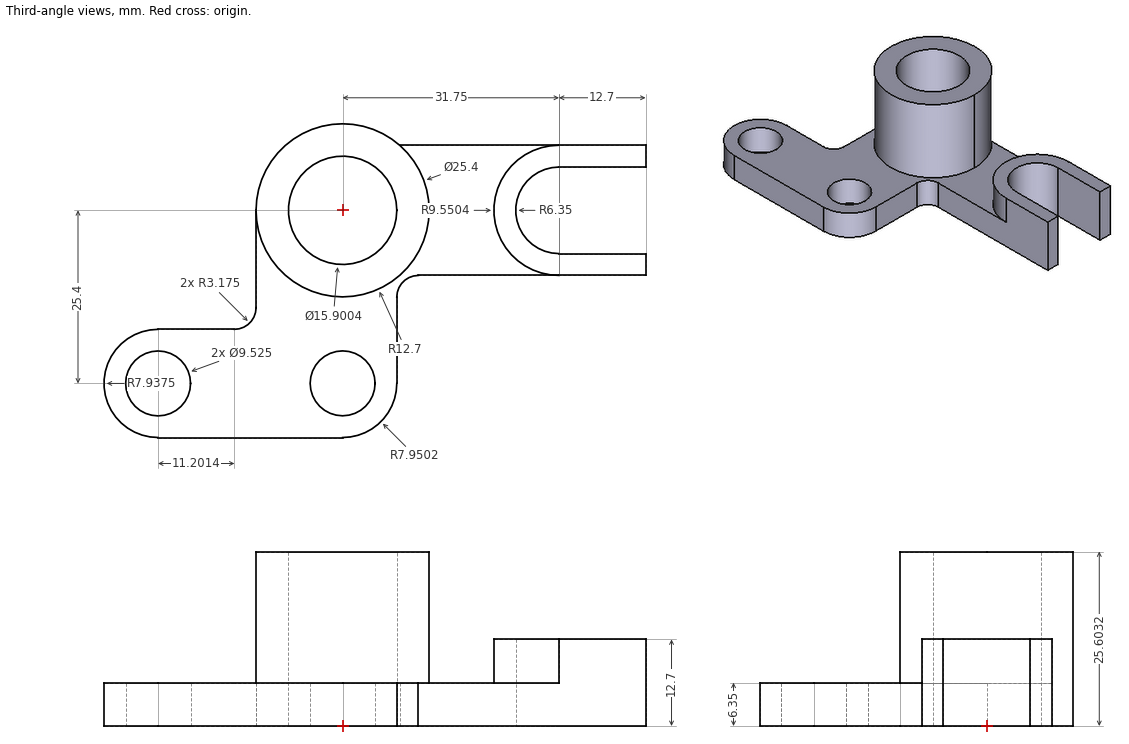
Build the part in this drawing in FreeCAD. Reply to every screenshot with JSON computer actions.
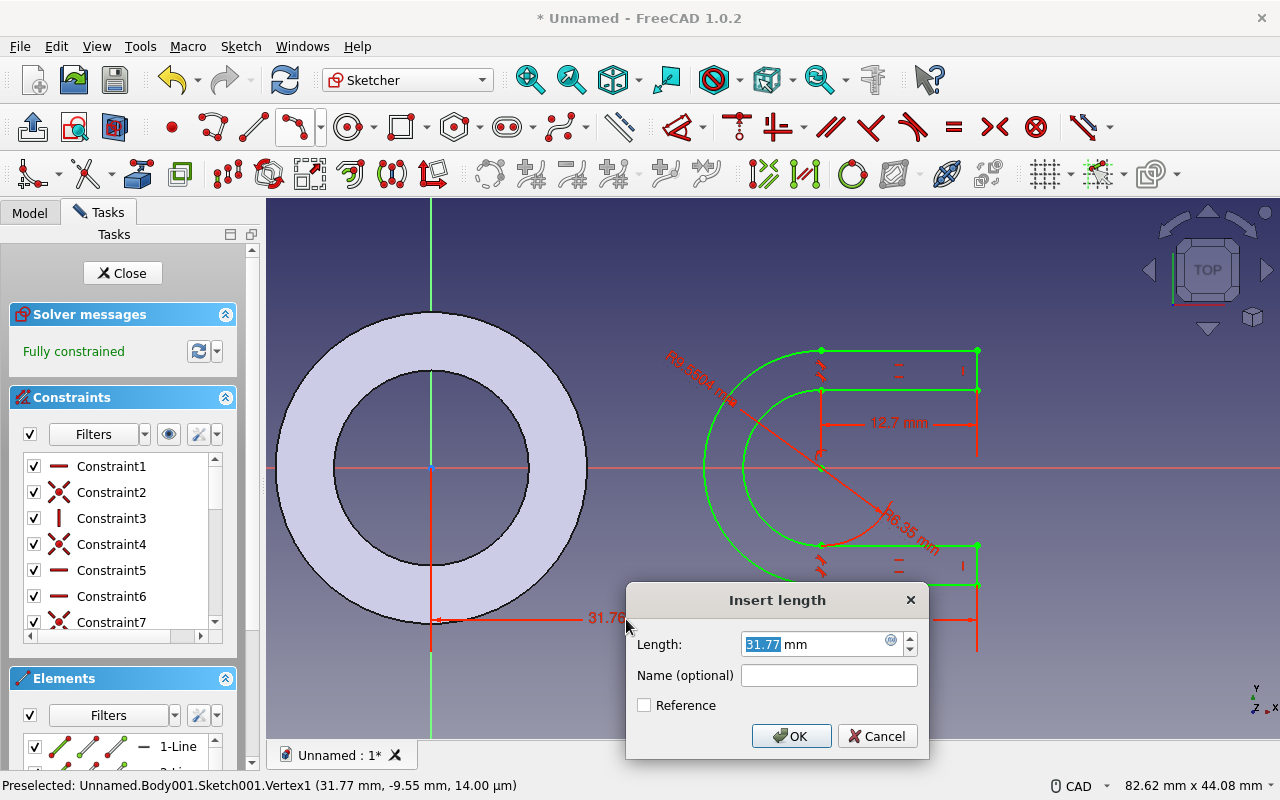
{"action": "type", "text": "31.75"}
{"action": "key", "text": "Return"}
{"action": "key", "text": "Escape"}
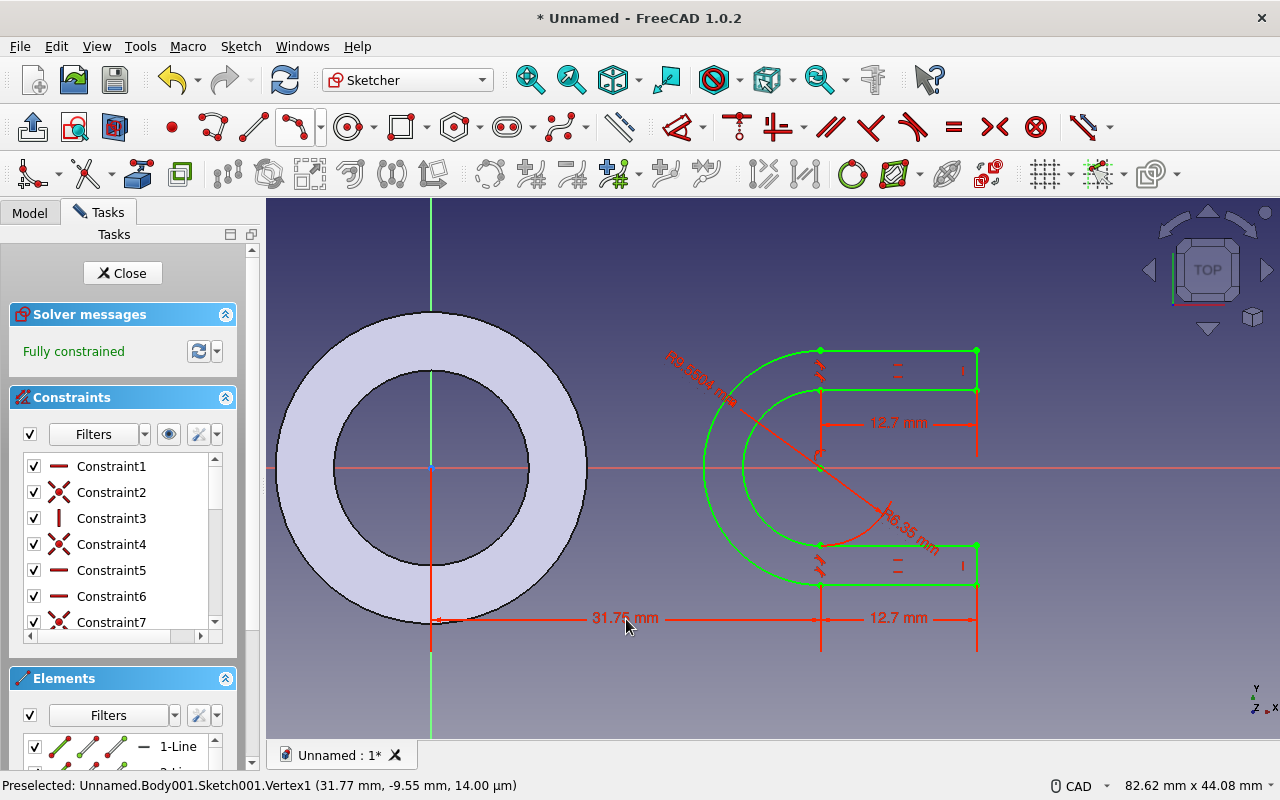
{"action": "left_click", "coordinate": [123, 273]}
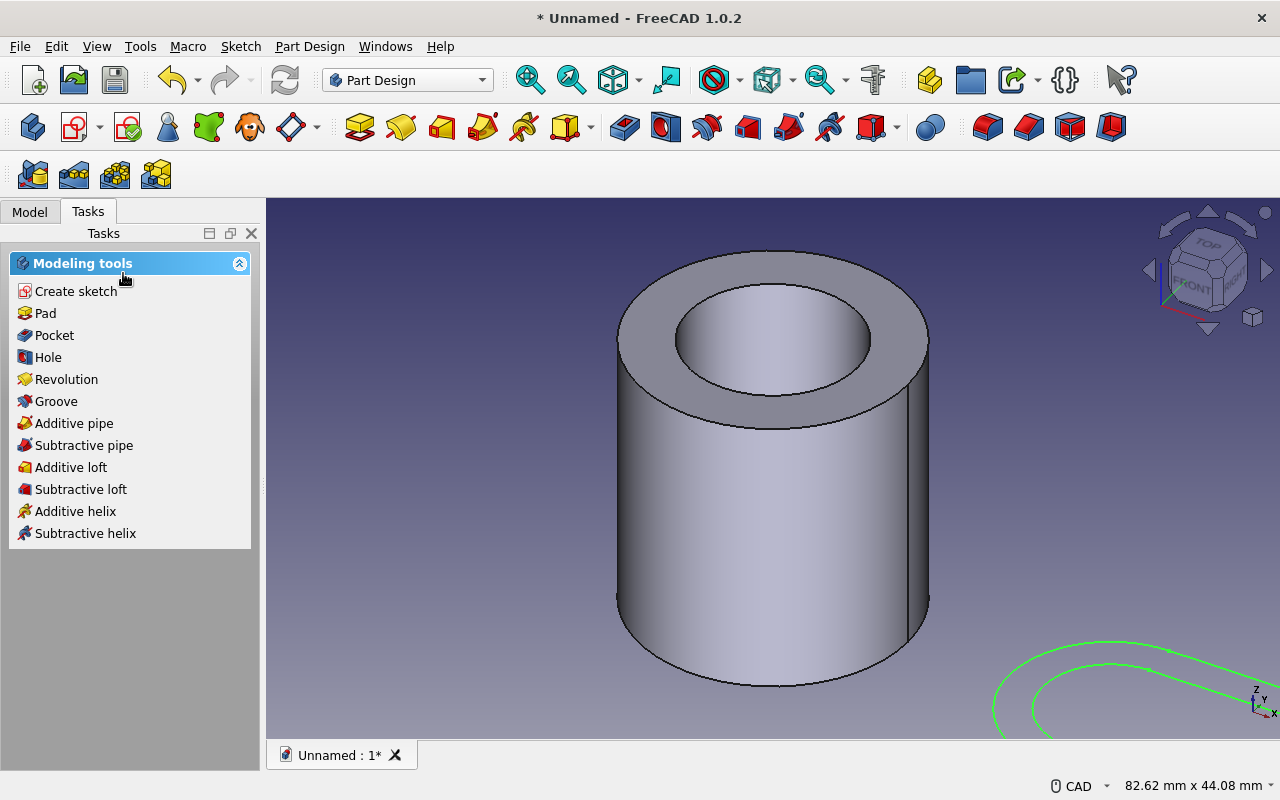
{"action": "left_click", "coordinate": [360, 128]}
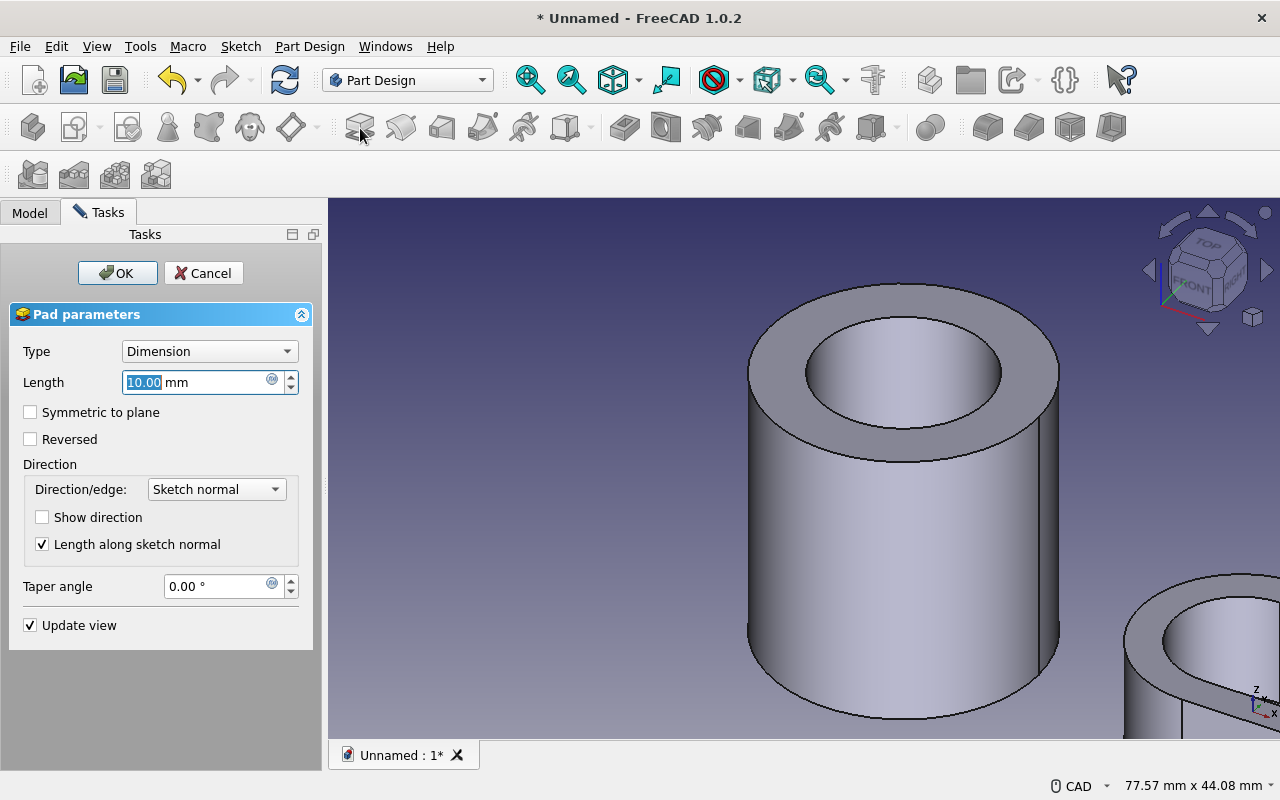
{"action": "type", "text": "12.7"}
{"action": "key", "text": "Tab"}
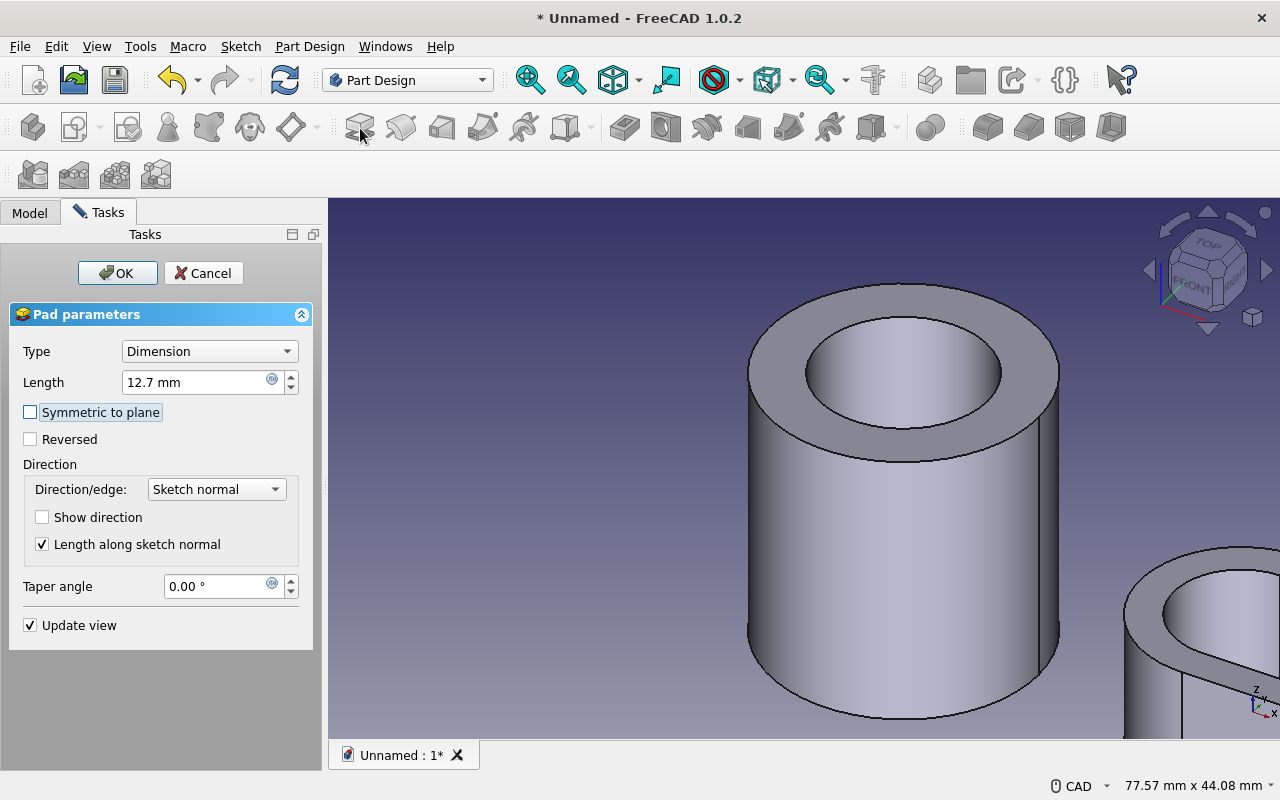
{"action": "left_click", "coordinate": [118, 273]}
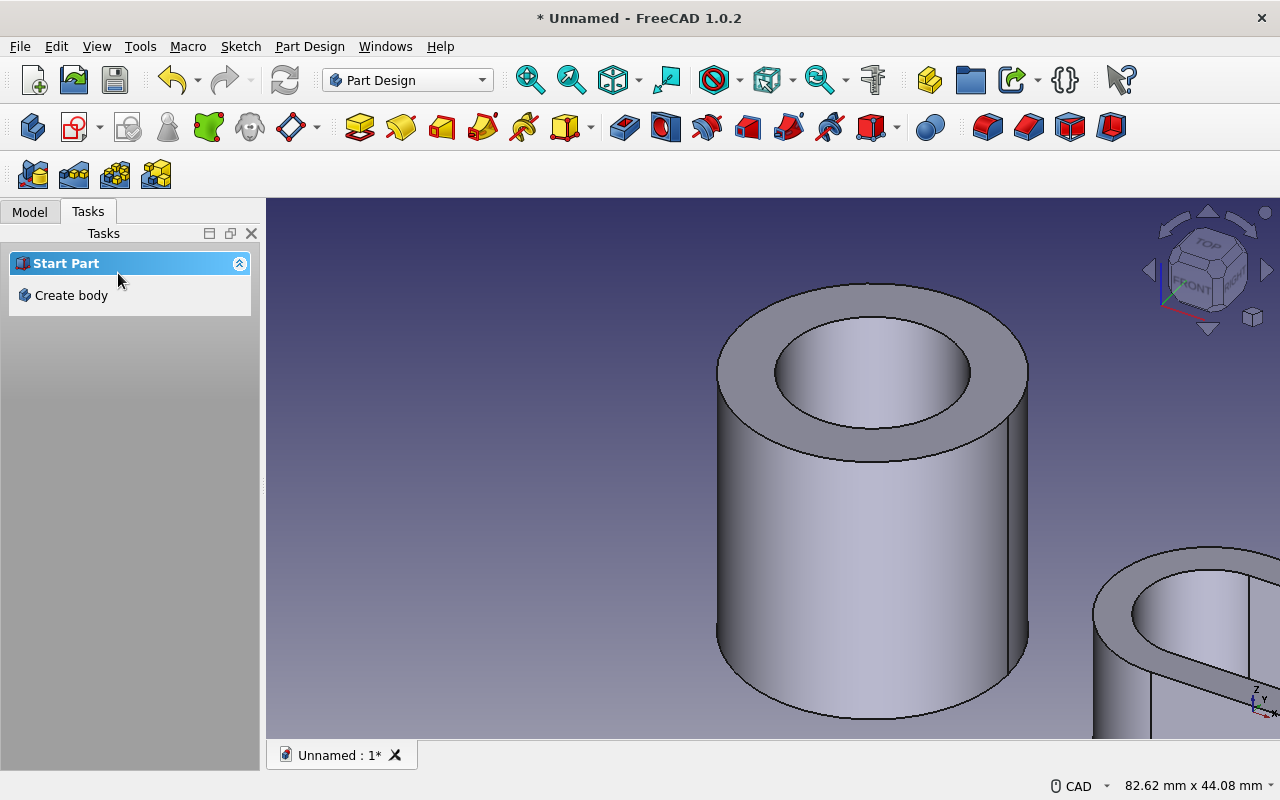
{"action": "left_click", "coordinate": [531, 80]}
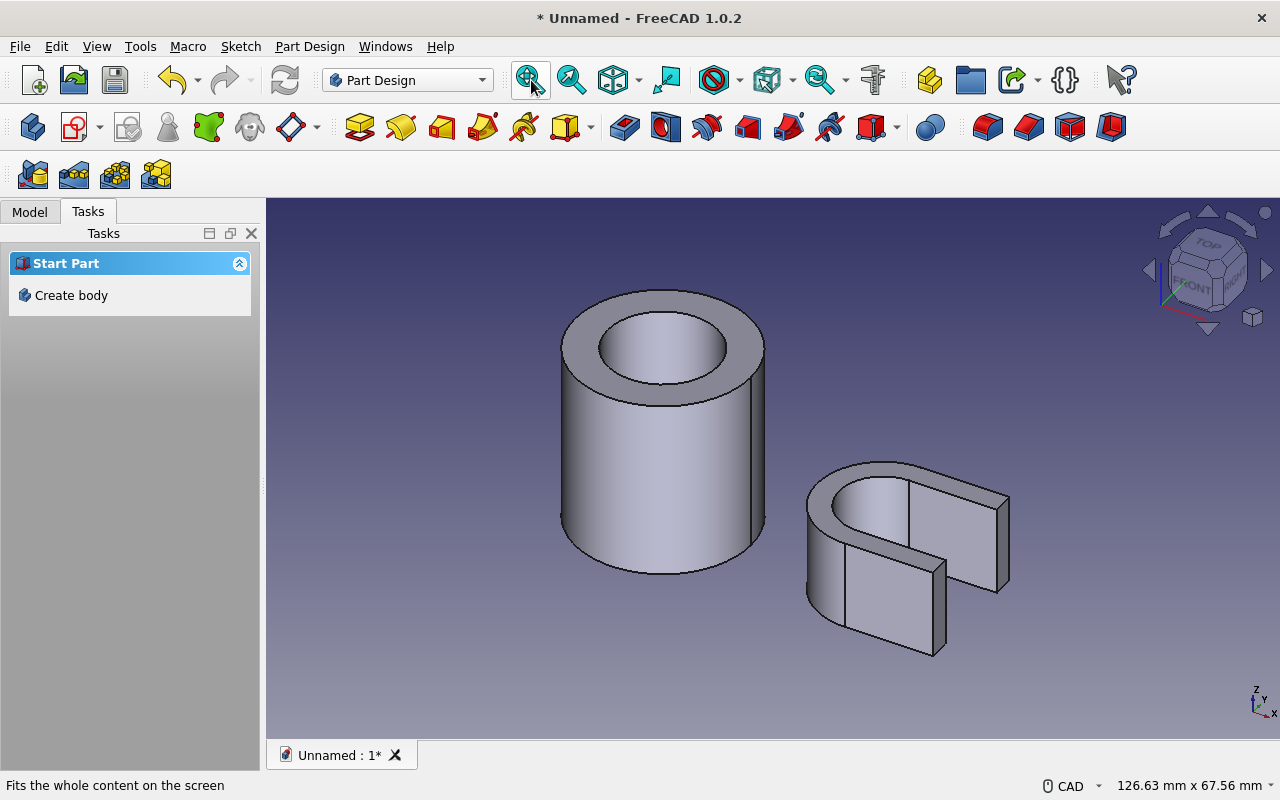
{"action": "left_click", "coordinate": [30, 212]}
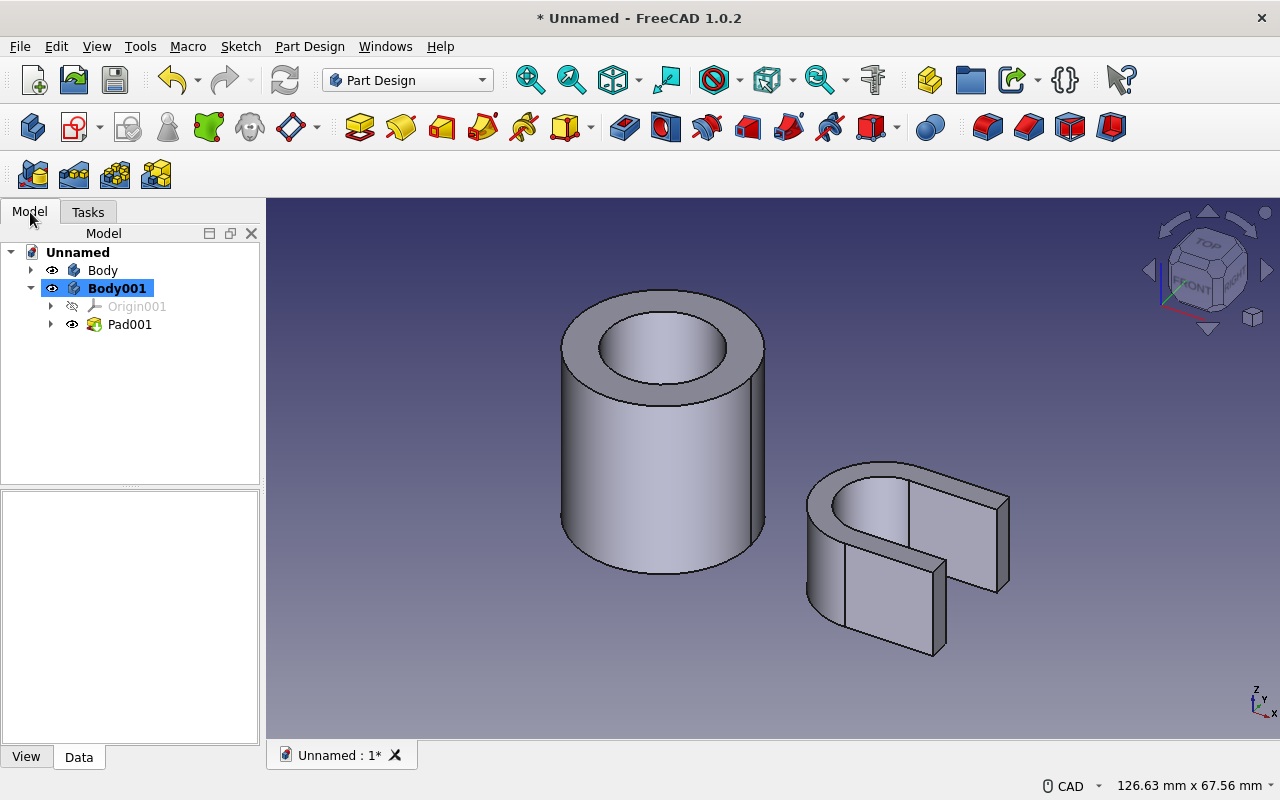
{"action": "double_click", "coordinate": [97, 270]}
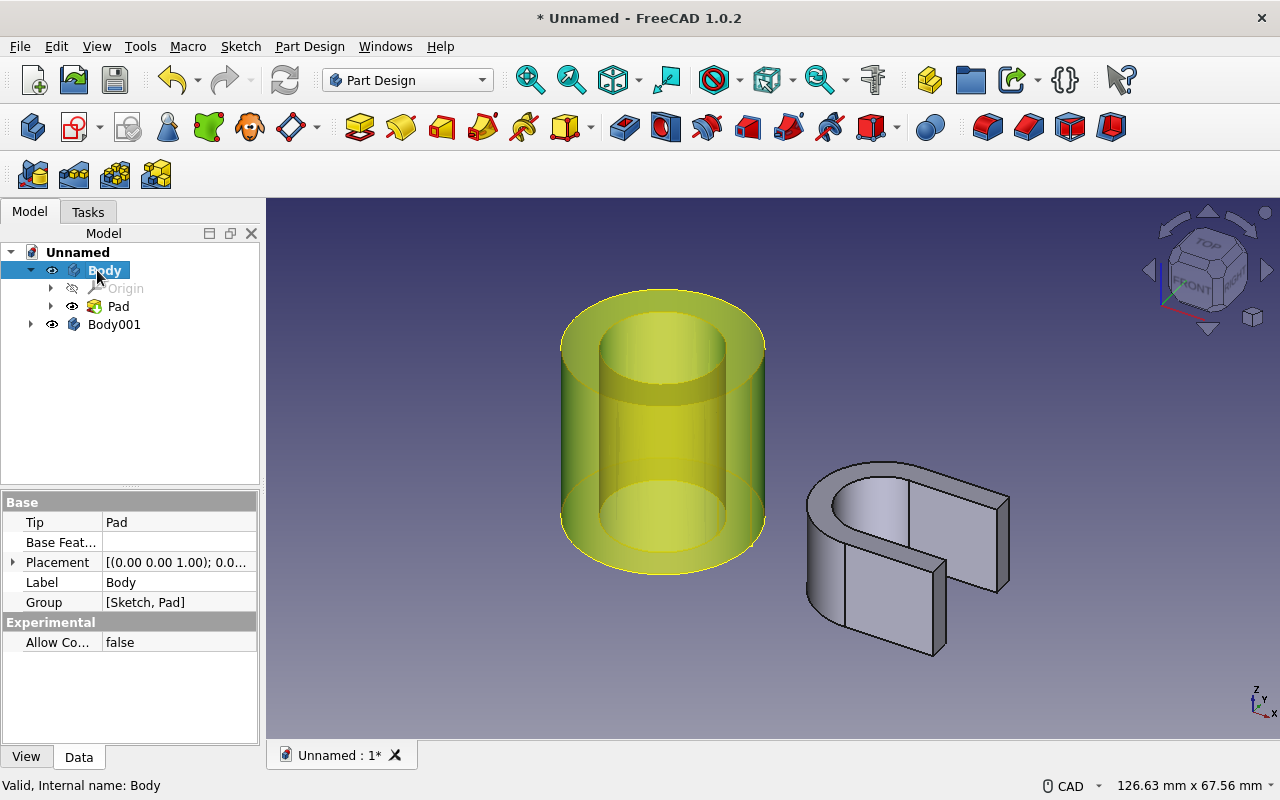
{"action": "left_click", "coordinate": [97, 270]}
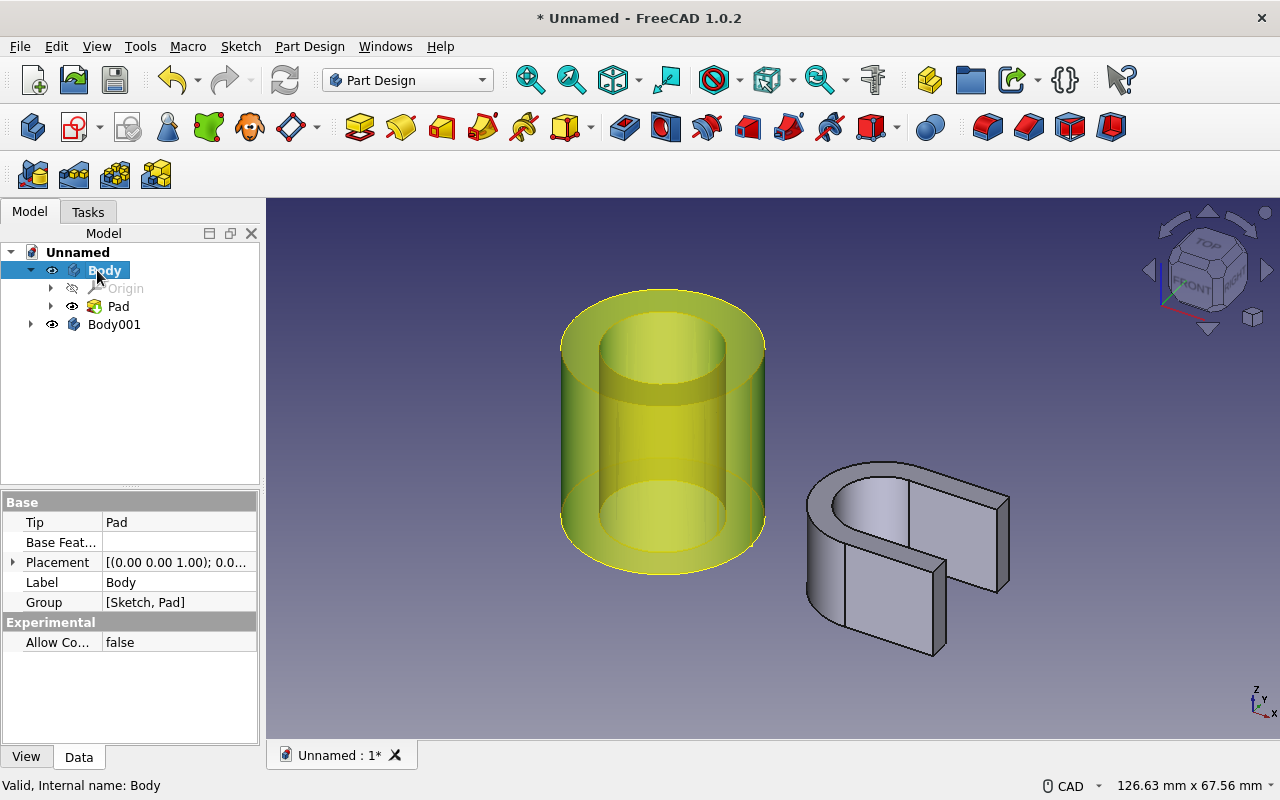
{"action": "left_click", "coordinate": [148, 642]}